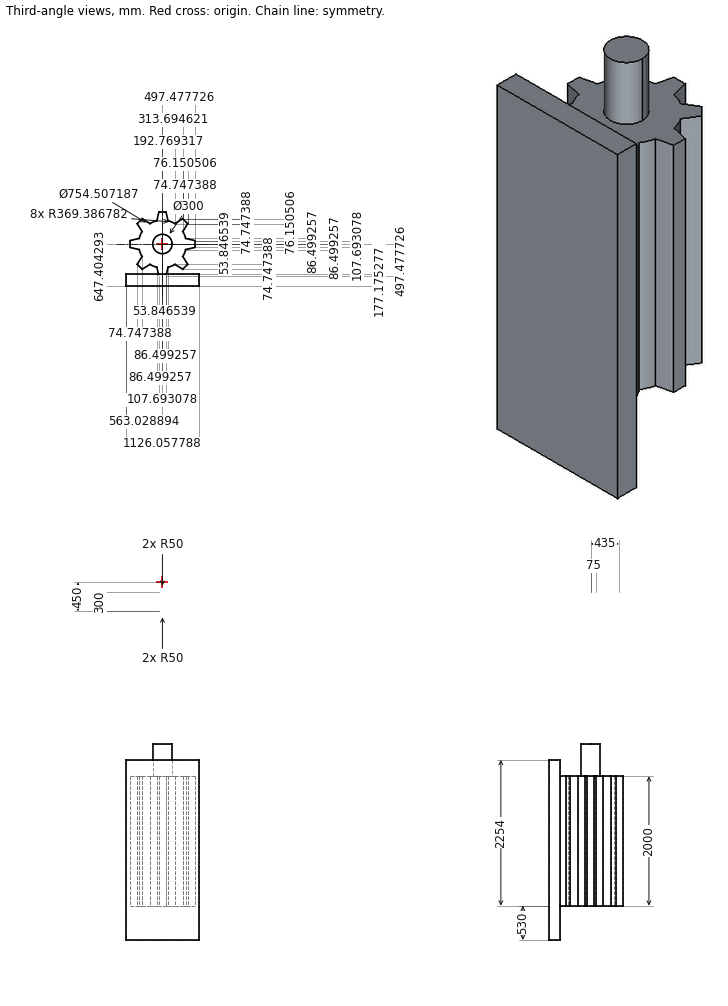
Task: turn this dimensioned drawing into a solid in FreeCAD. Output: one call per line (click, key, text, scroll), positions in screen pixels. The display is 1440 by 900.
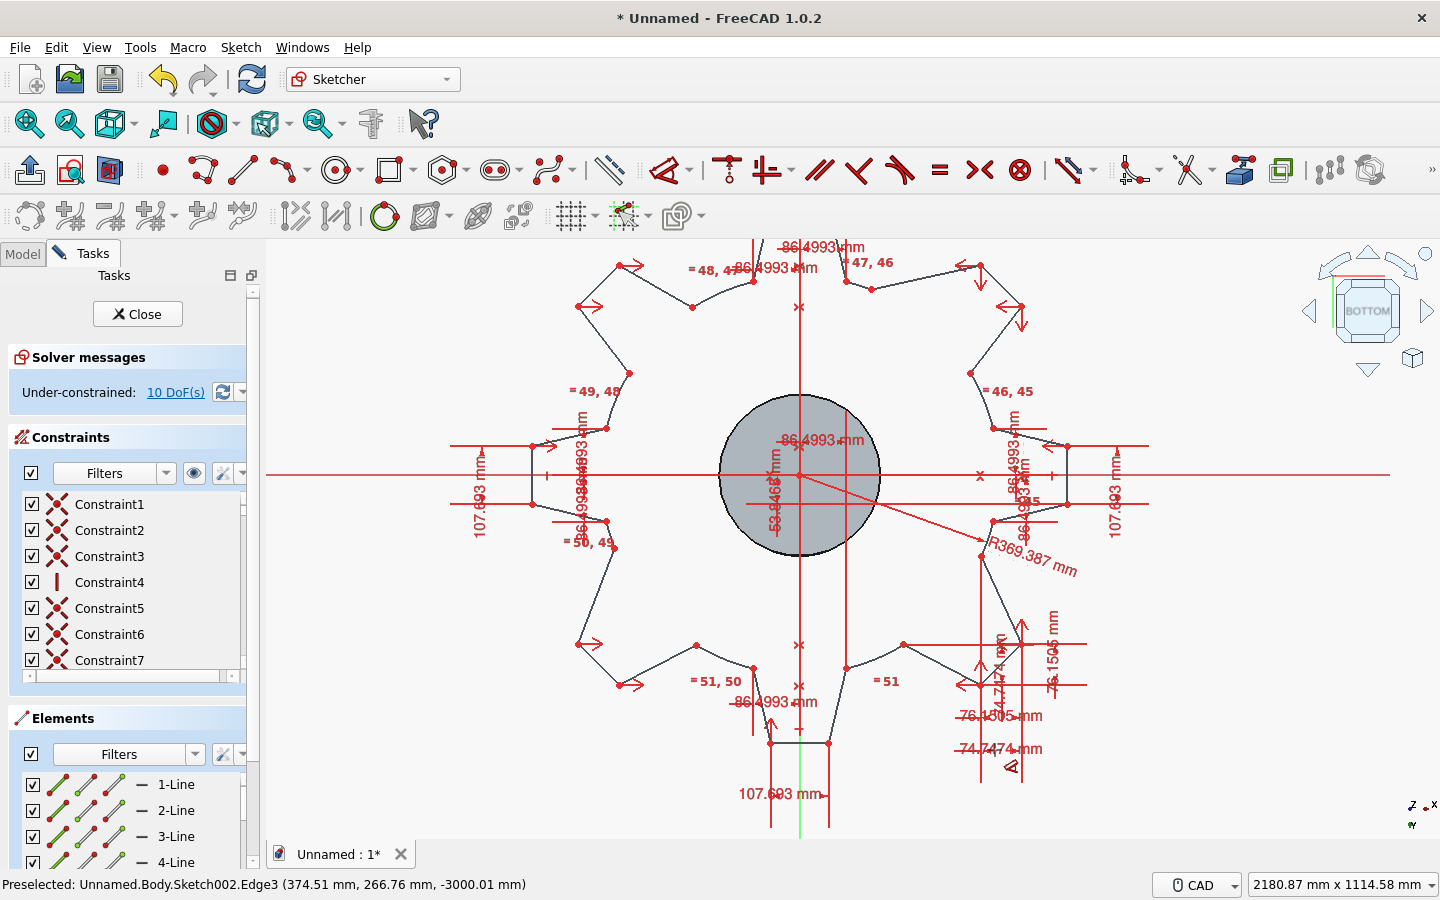
click(986, 353)
click(1008, 273)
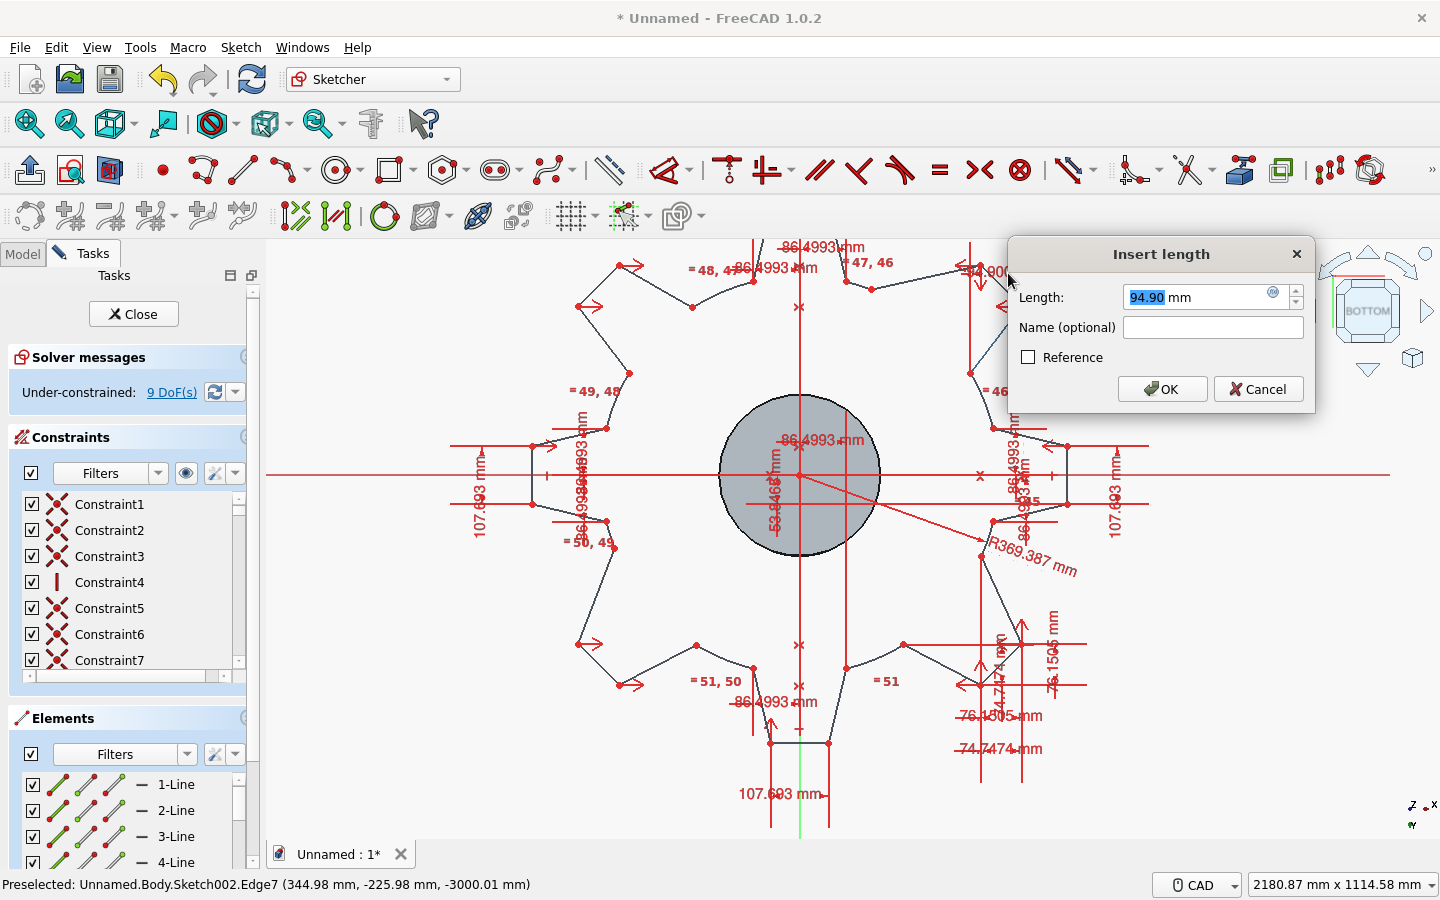
text(74.747388)
key(Return)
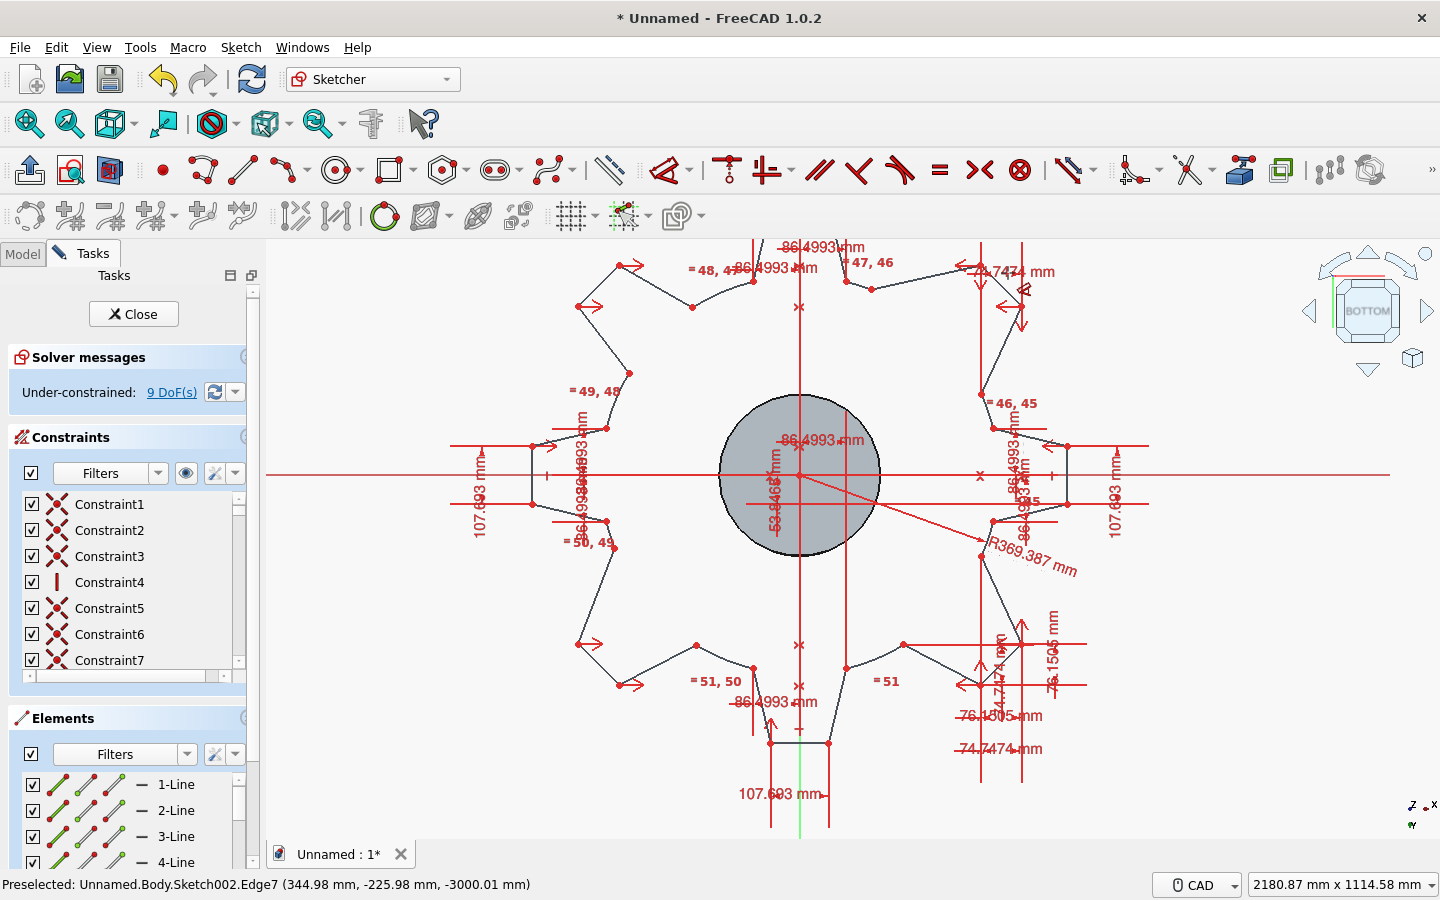
click(948, 273)
click(1087, 278)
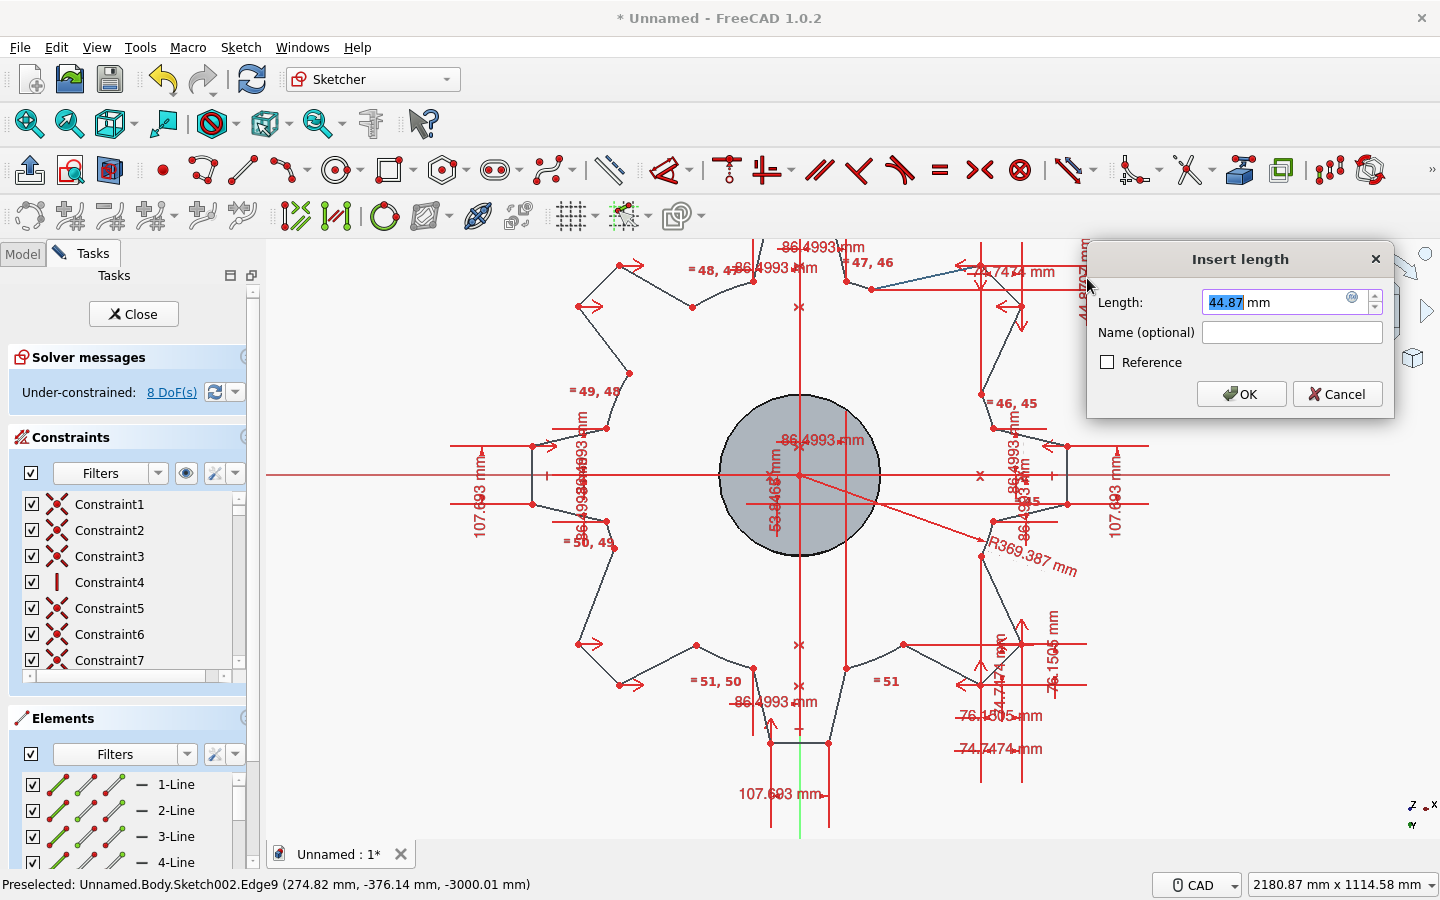
text(74.747388)
key(Return)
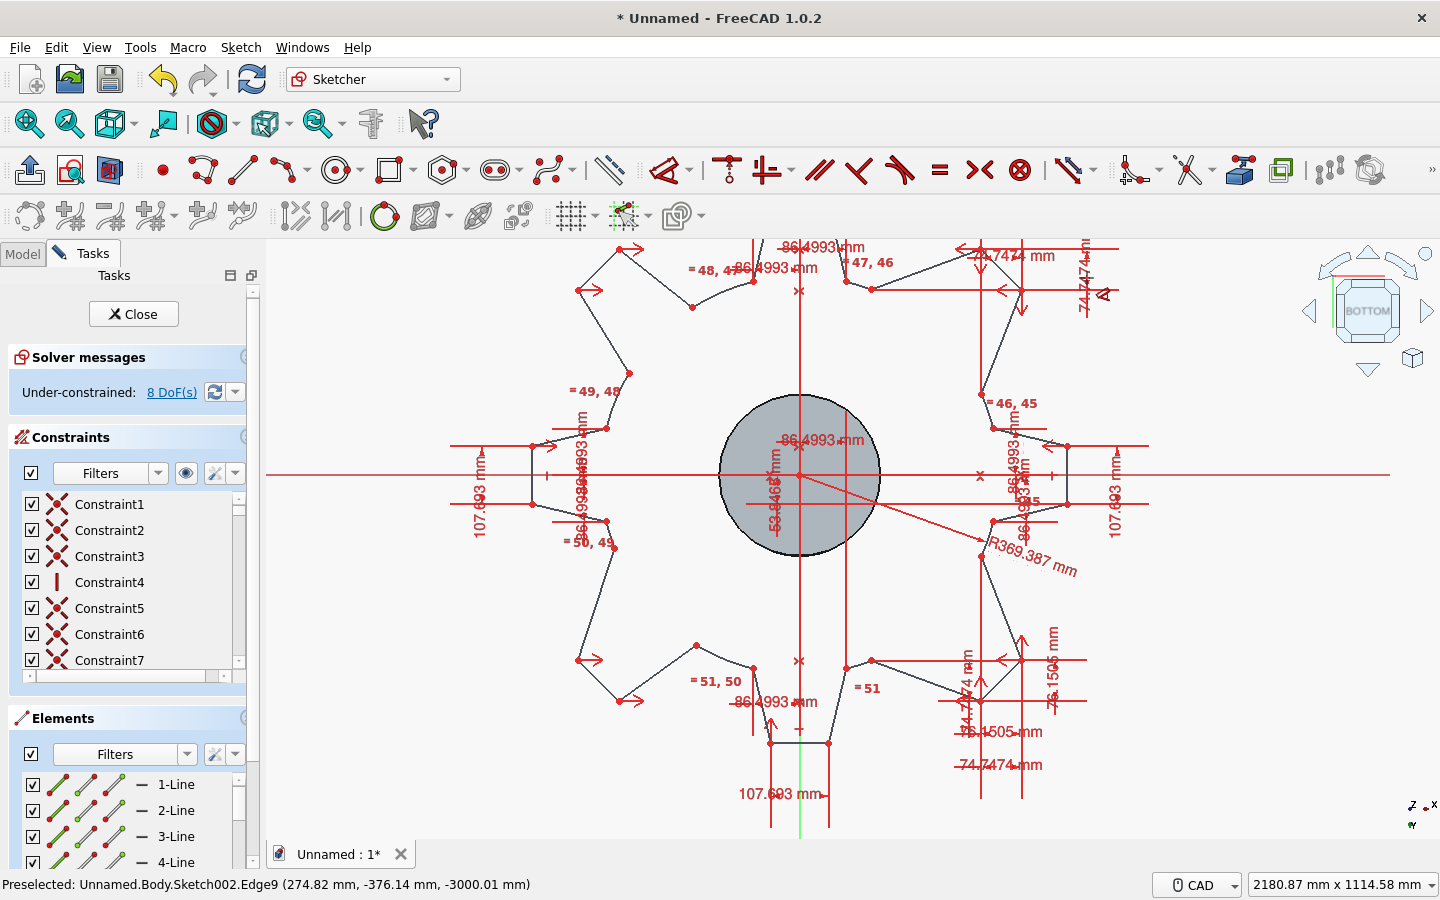
click(670, 290)
click(561, 287)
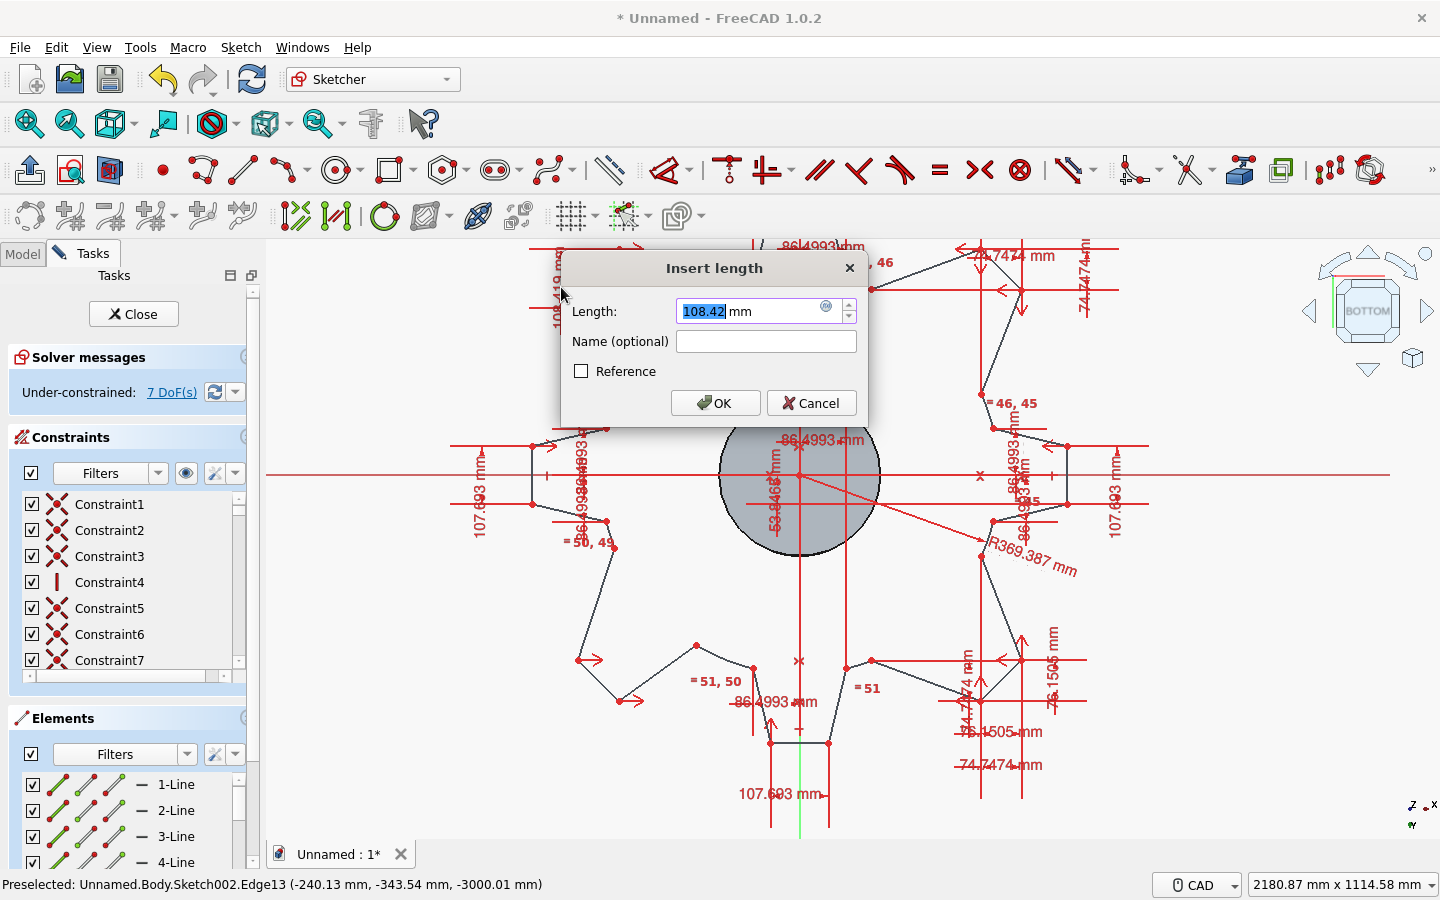
text(74.747388)
key(Return)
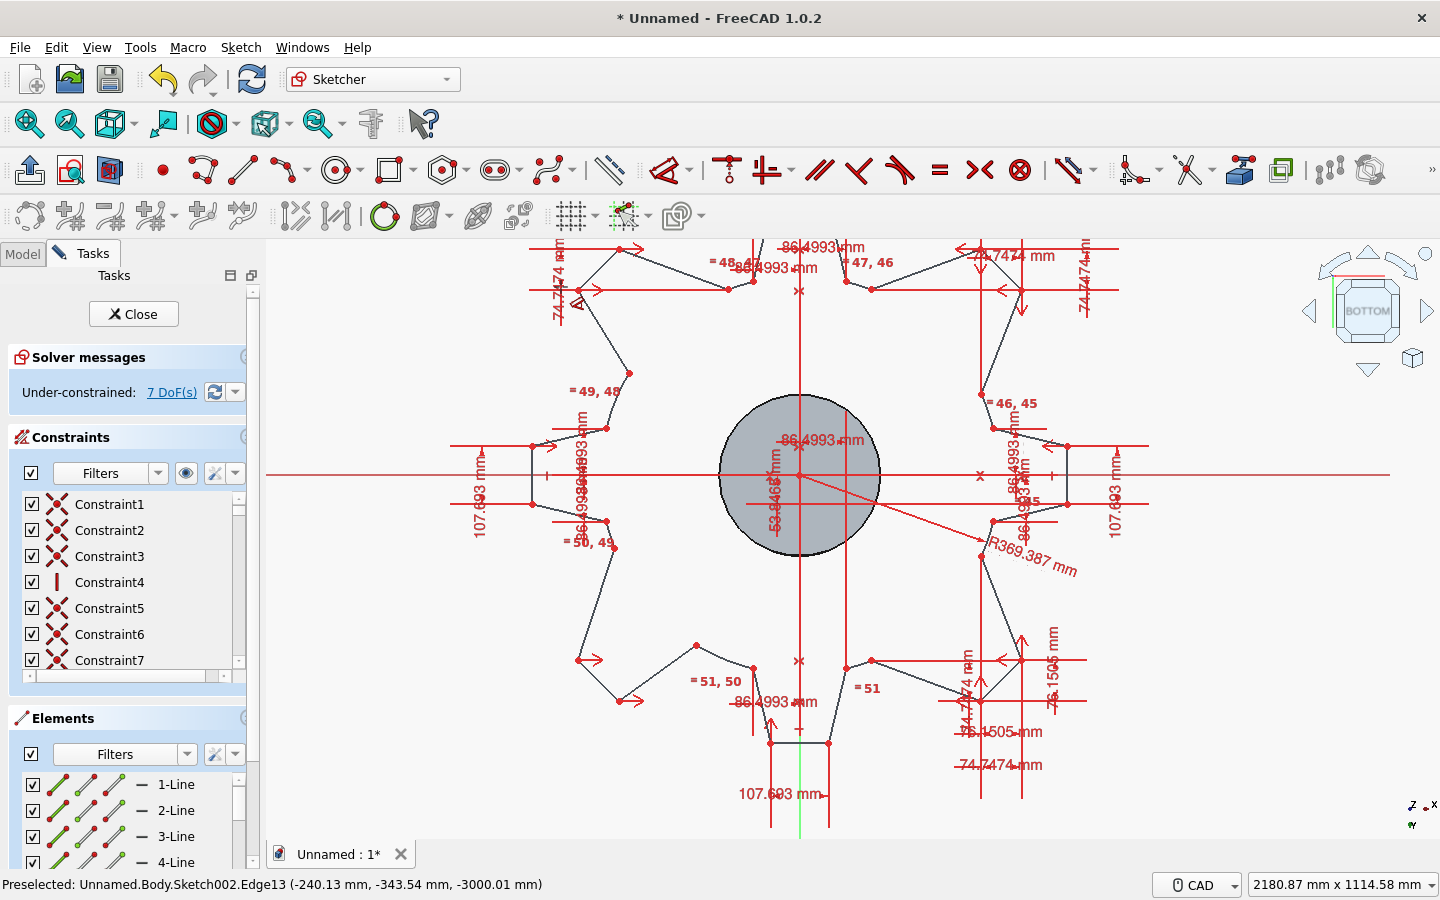
click(593, 315)
click(592, 407)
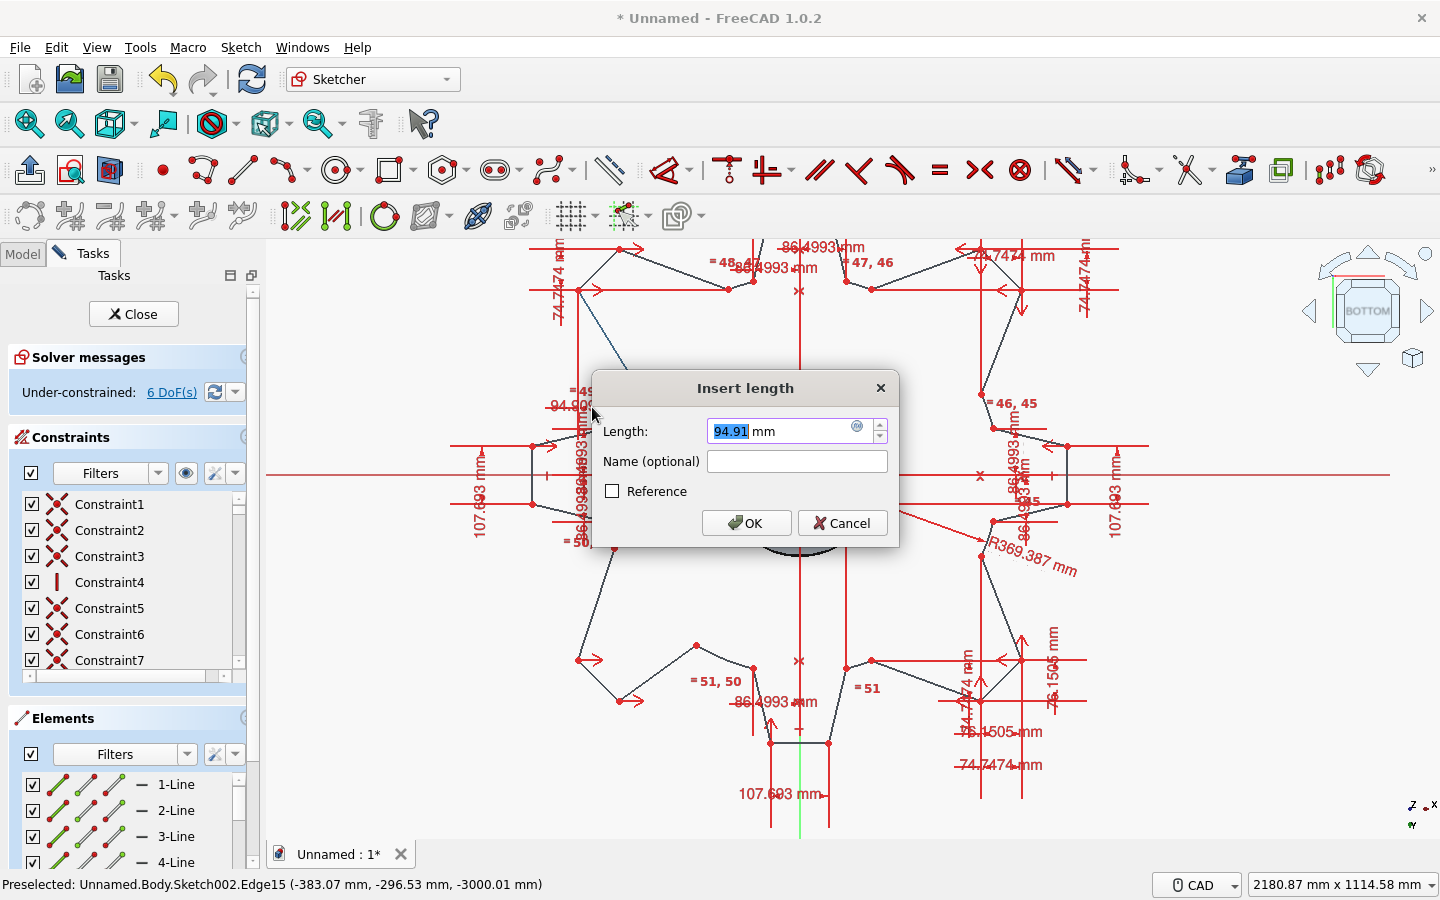
text(74.747388)
key(Return)